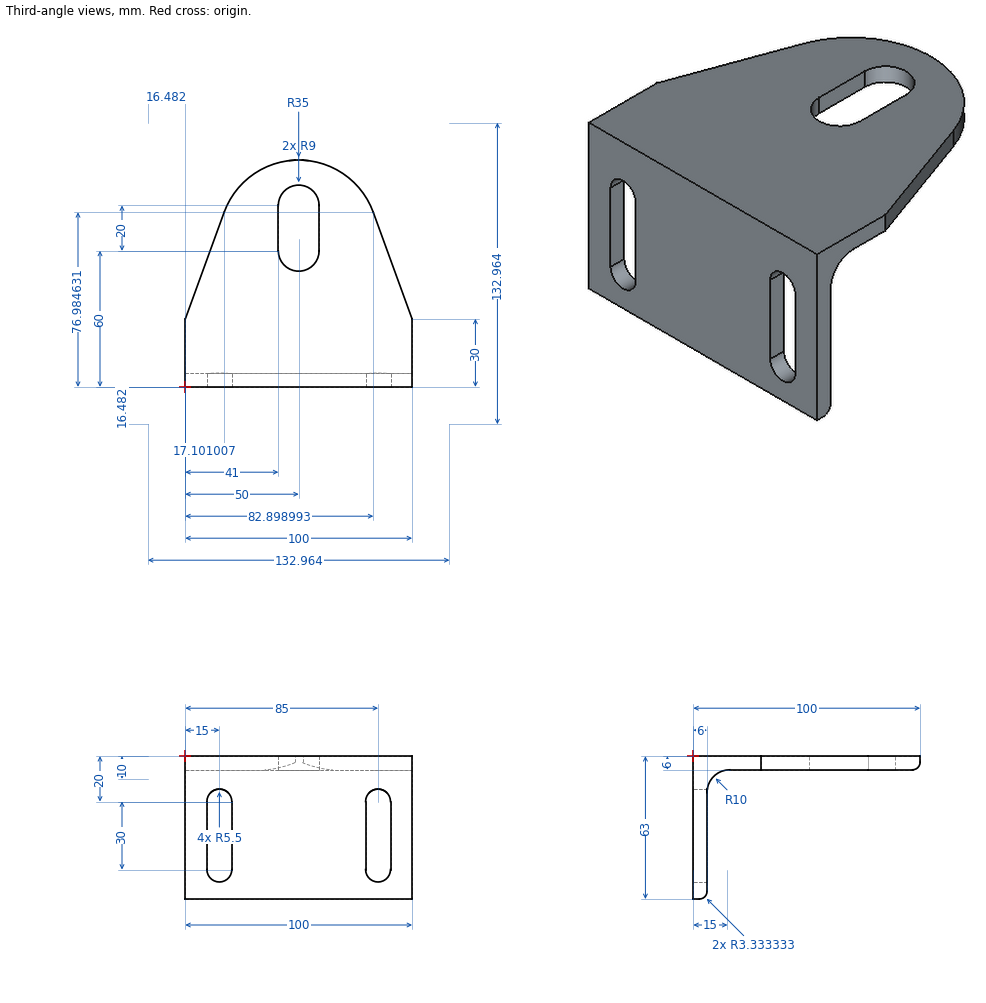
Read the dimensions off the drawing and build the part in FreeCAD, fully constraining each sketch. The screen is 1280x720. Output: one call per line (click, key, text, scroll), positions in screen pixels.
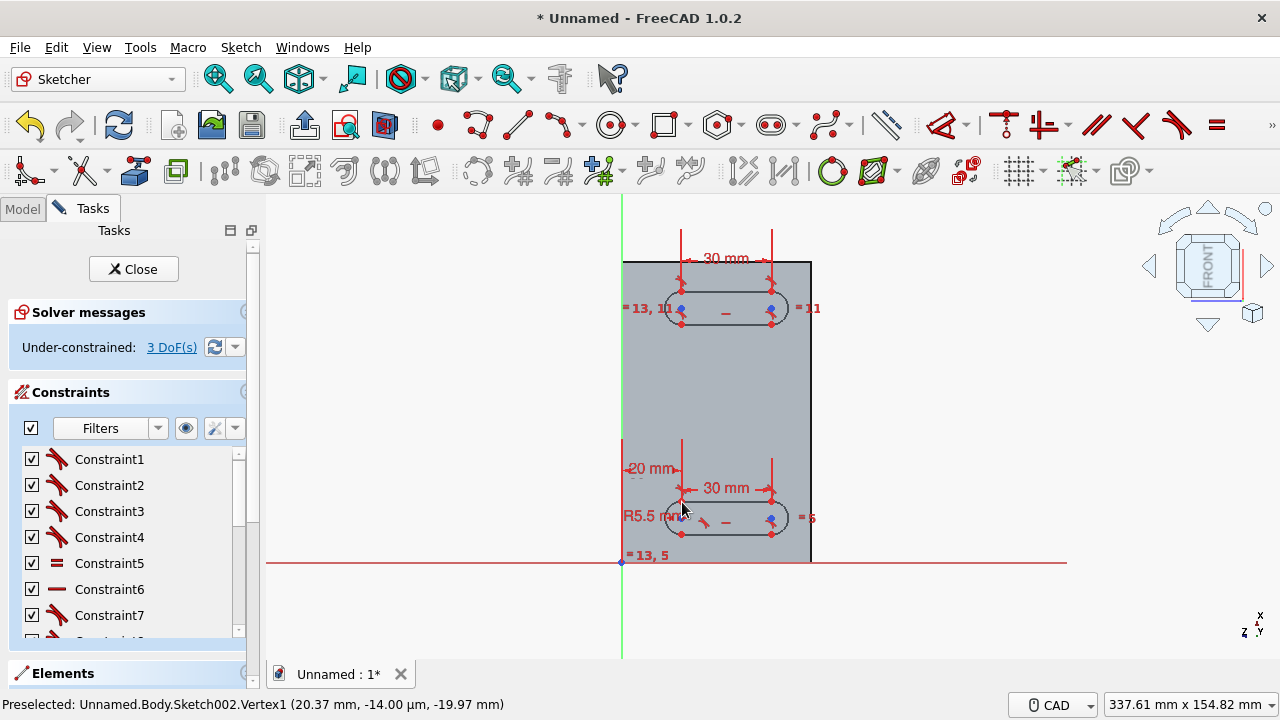
click(681, 292)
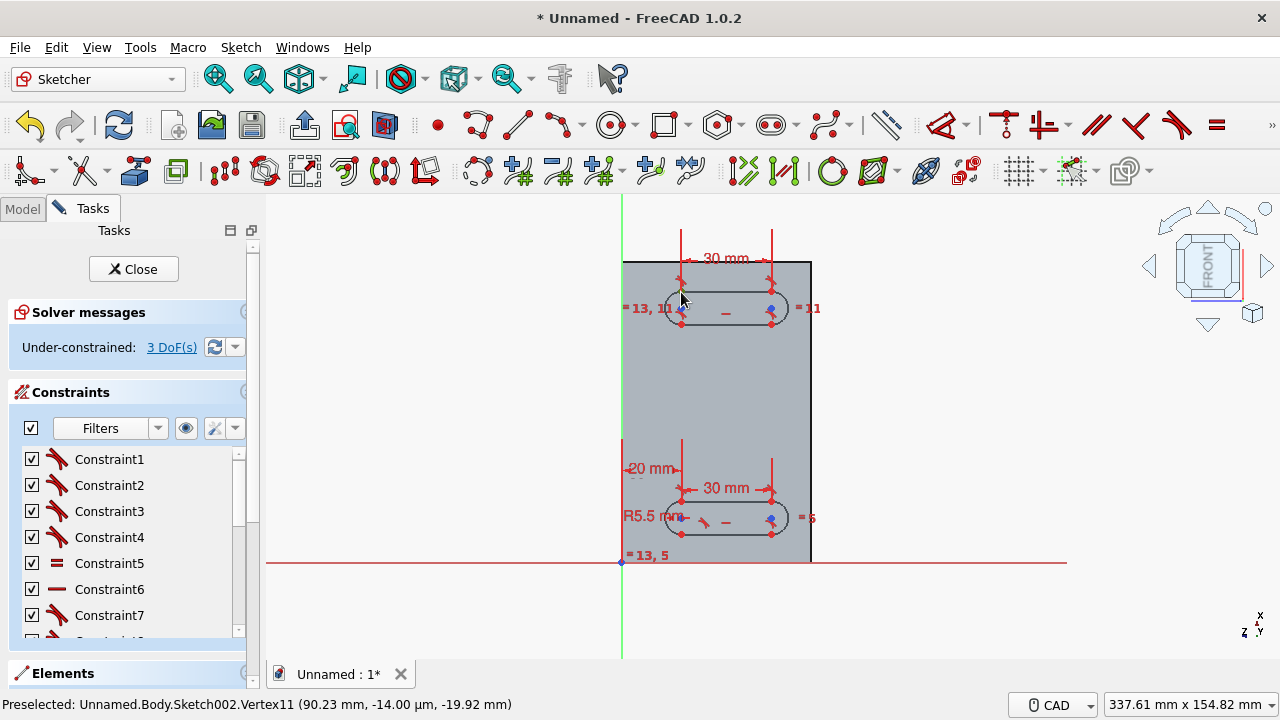
key(l)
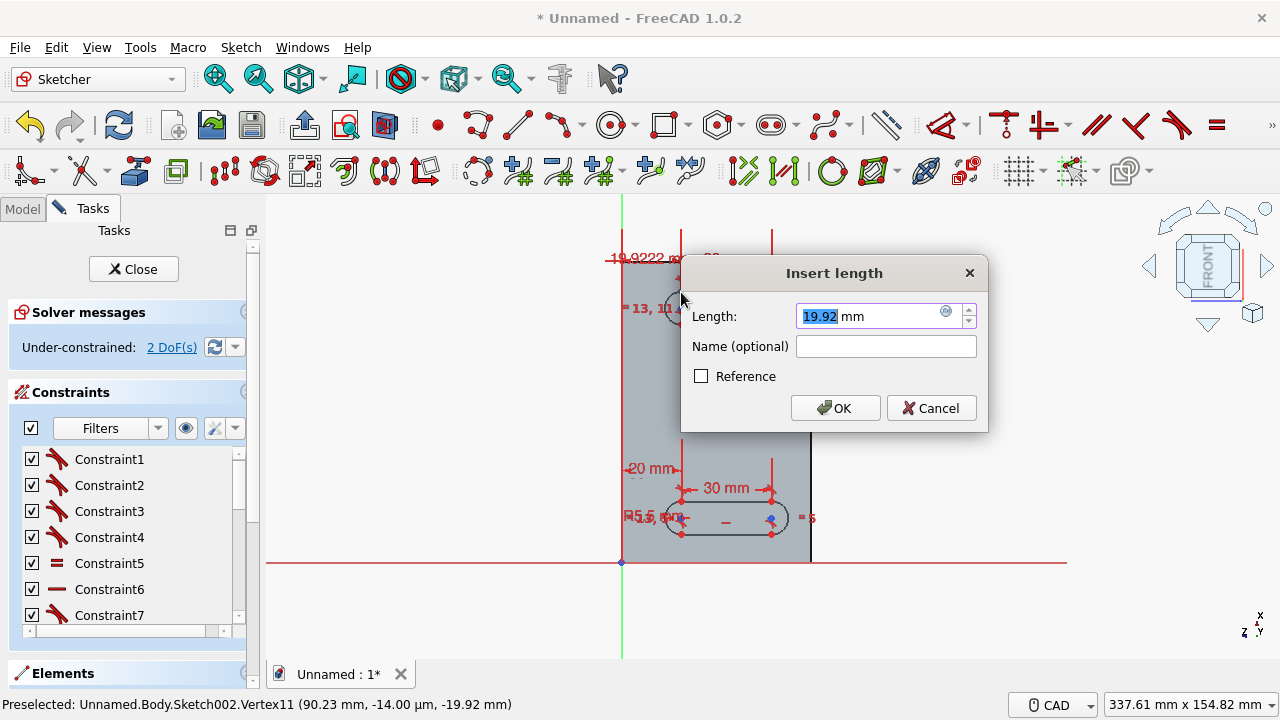
text(20)
key(Return)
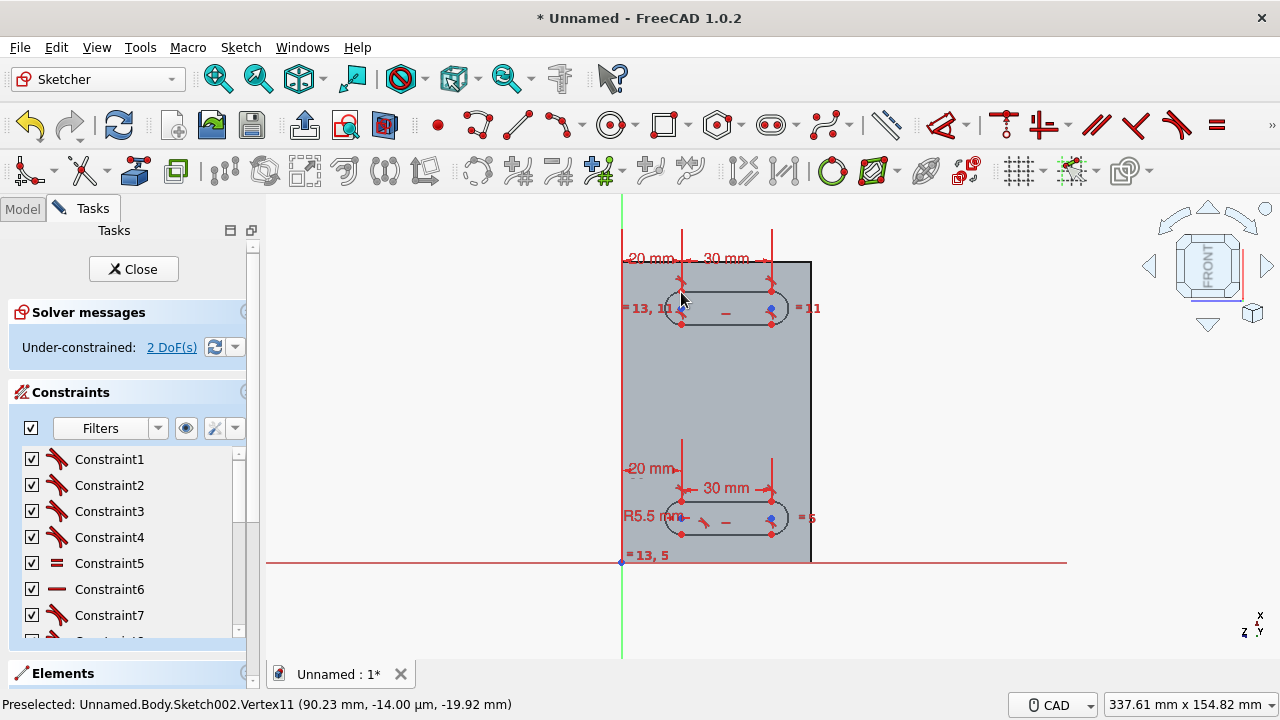
click(682, 518)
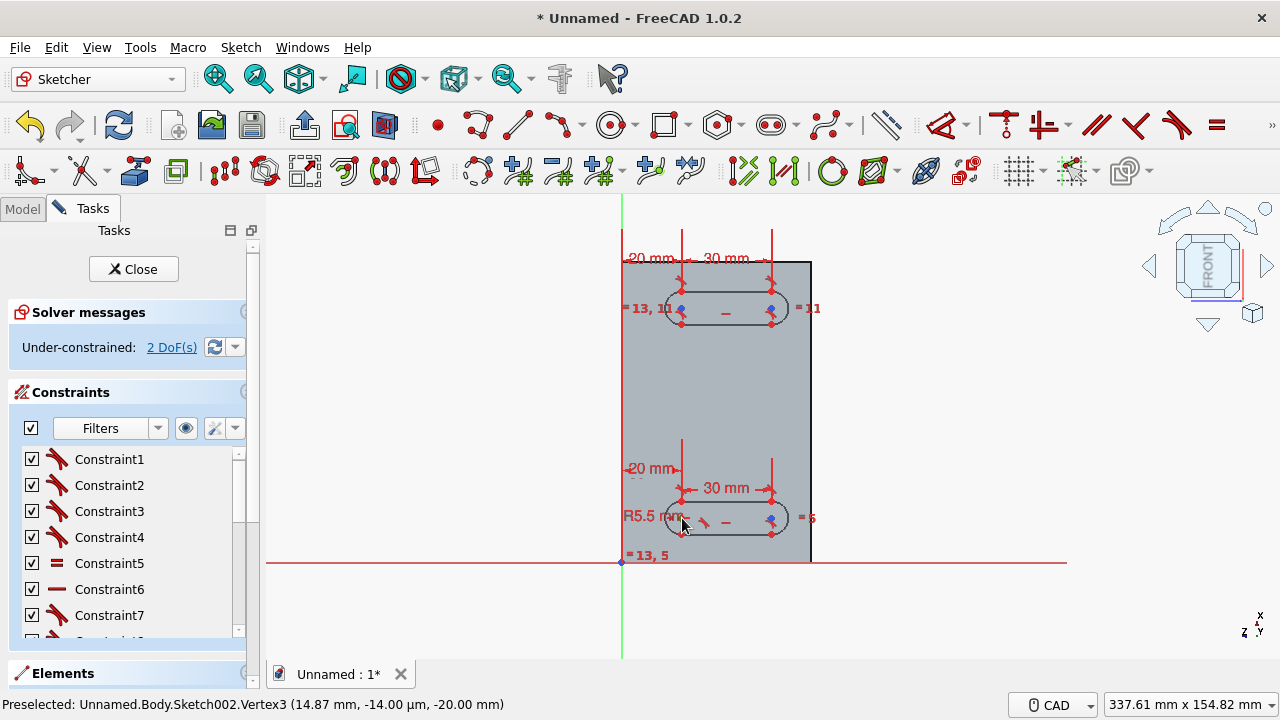
key(i)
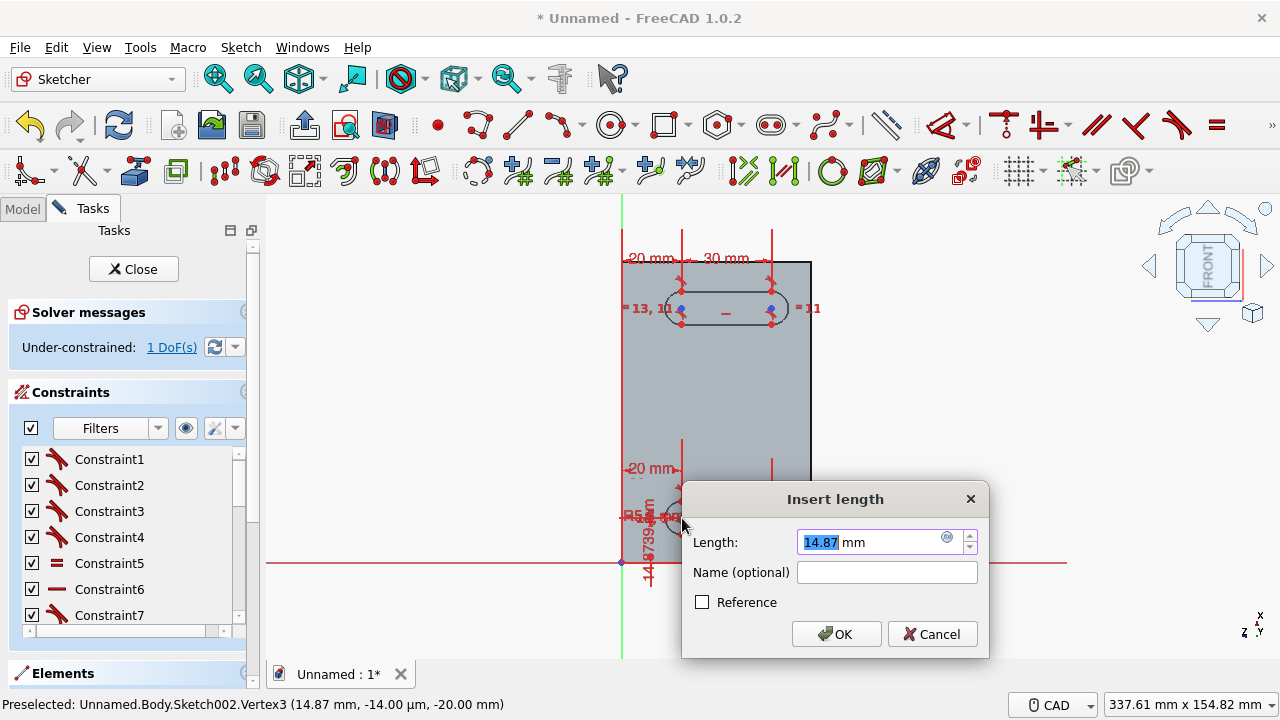
text(15)
key(Return)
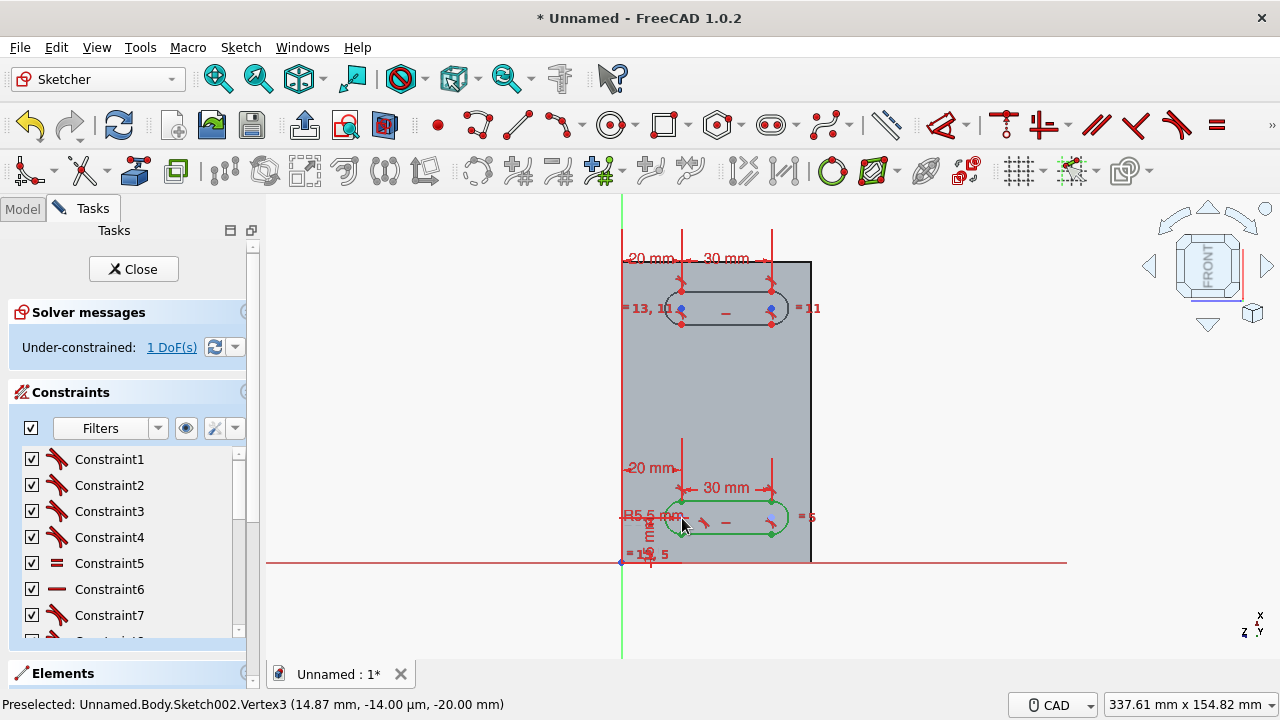
click(682, 308)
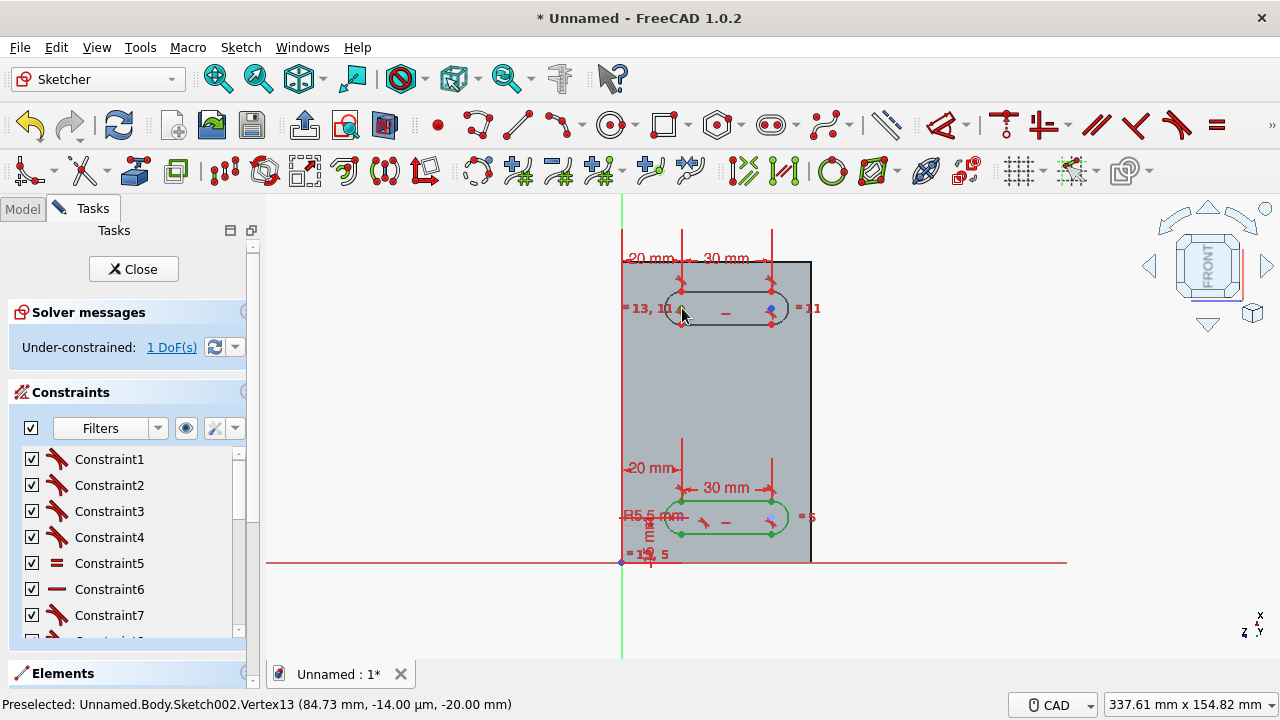
click(968, 126)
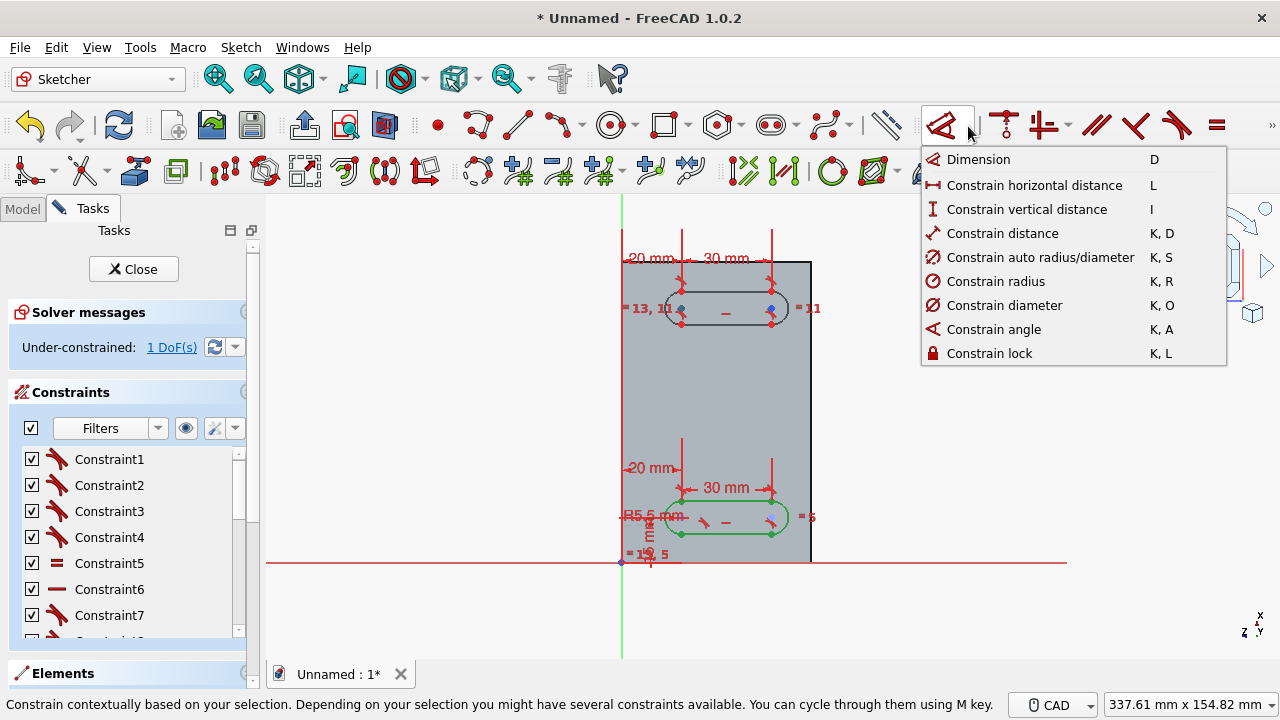
click(1074, 209)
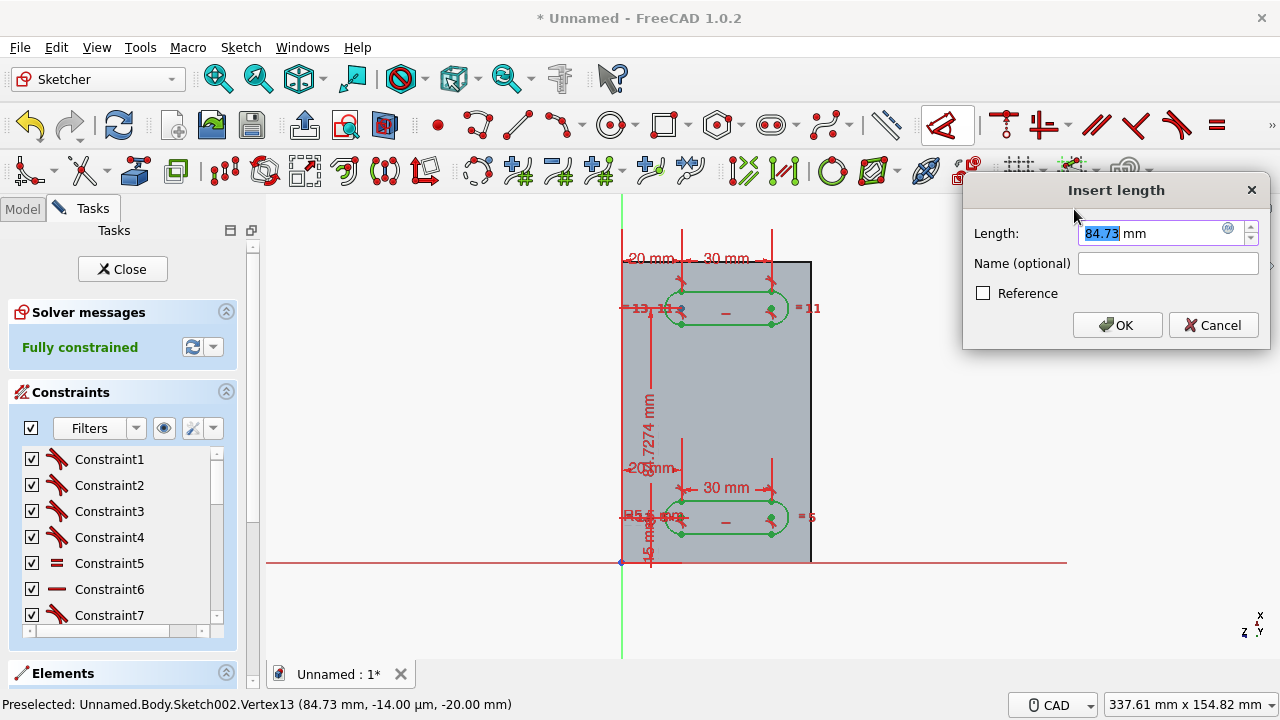
text(85)
key(Return)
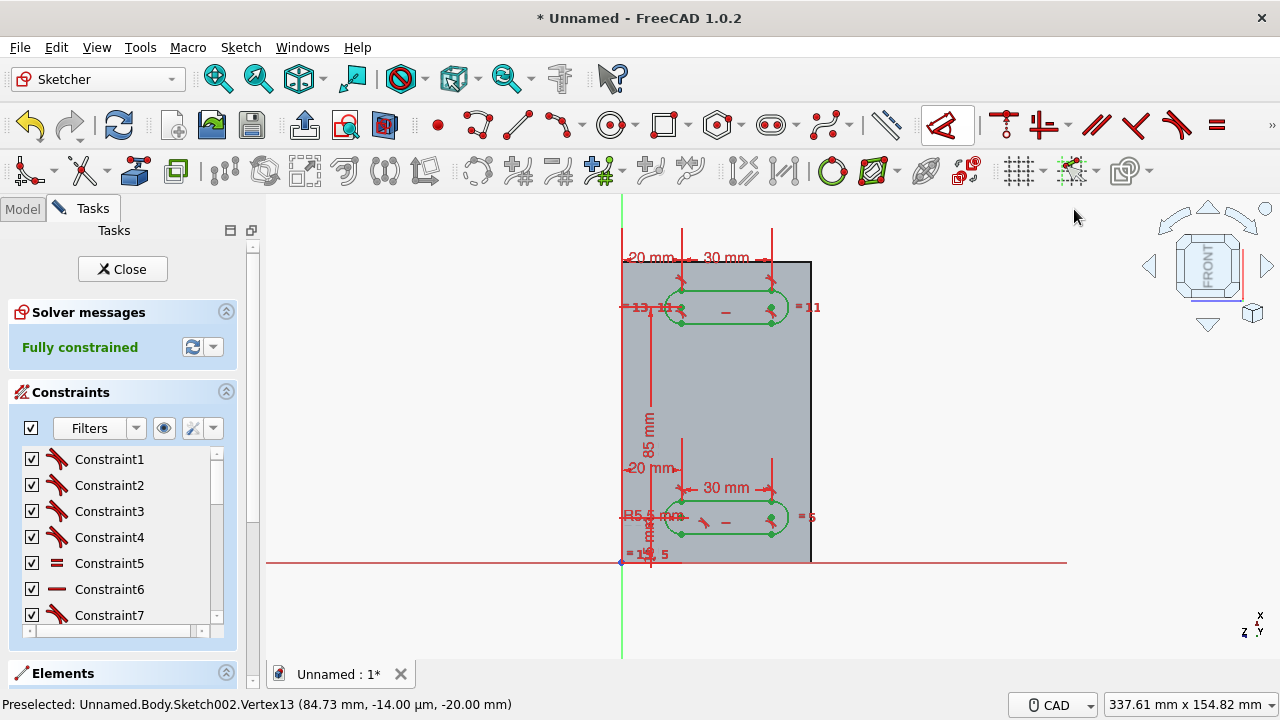
click(123, 269)